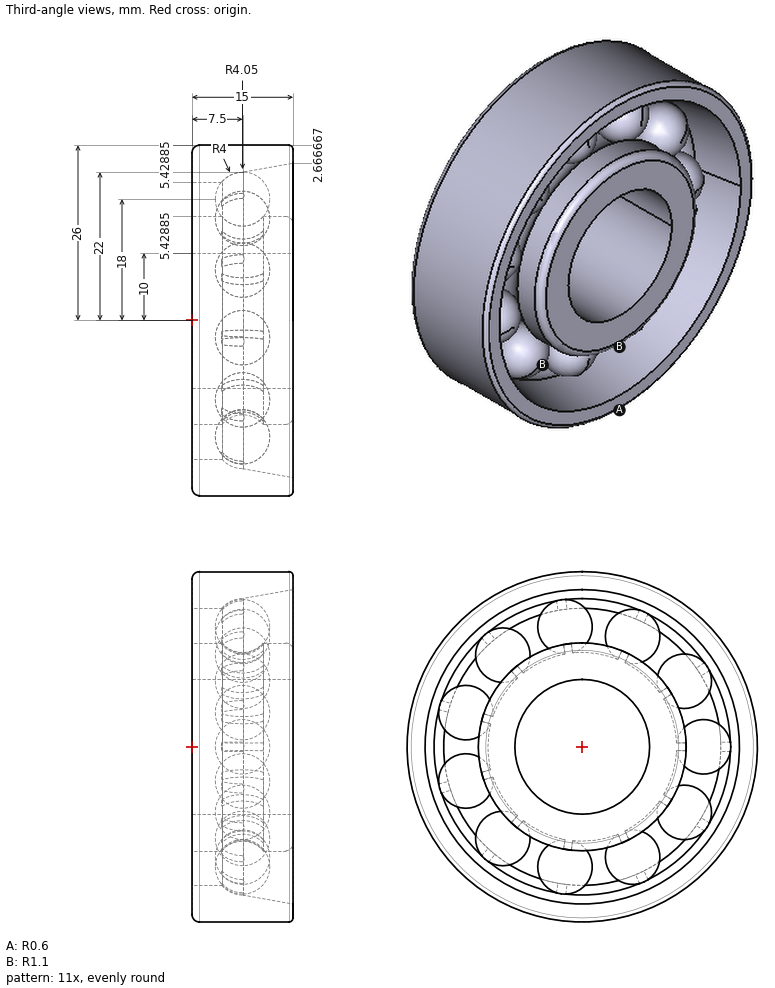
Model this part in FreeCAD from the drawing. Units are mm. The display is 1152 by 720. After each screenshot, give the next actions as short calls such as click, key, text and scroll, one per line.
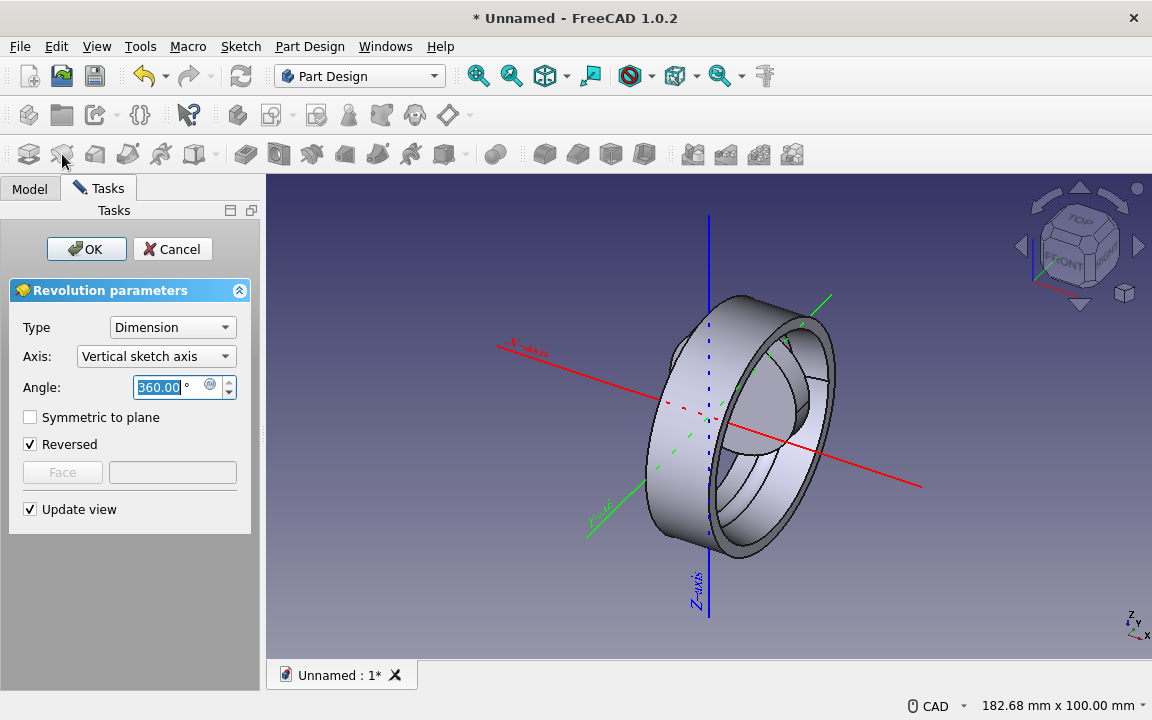
click(157, 356)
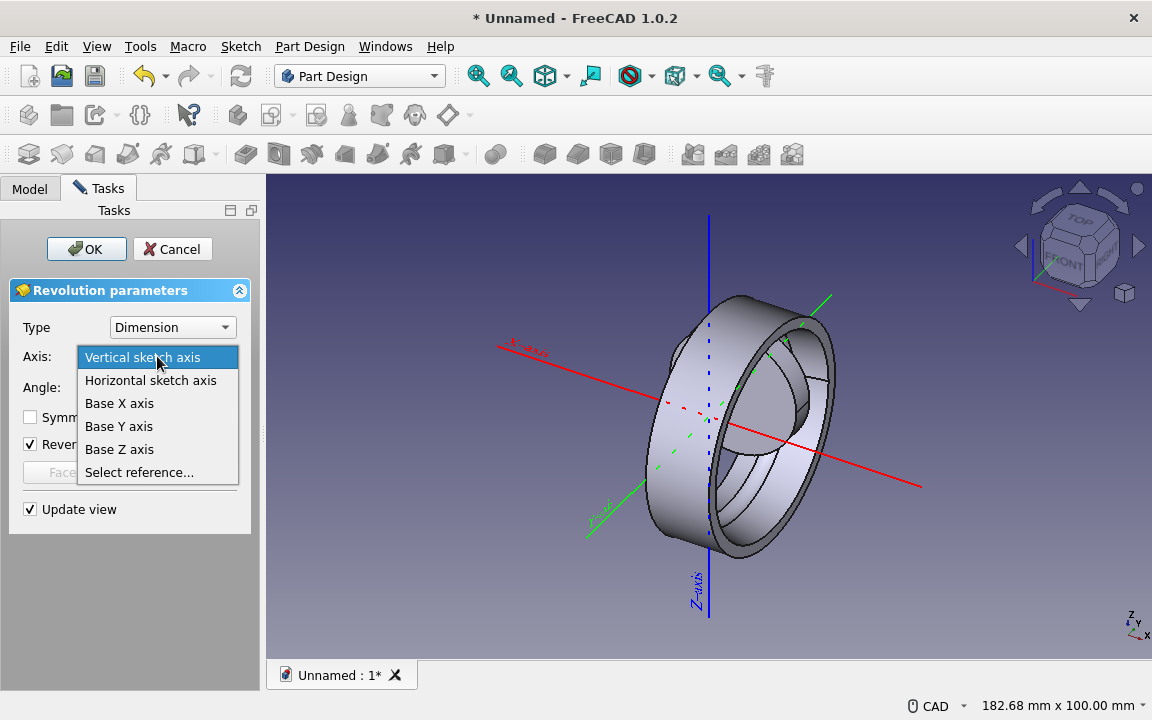
click(156, 380)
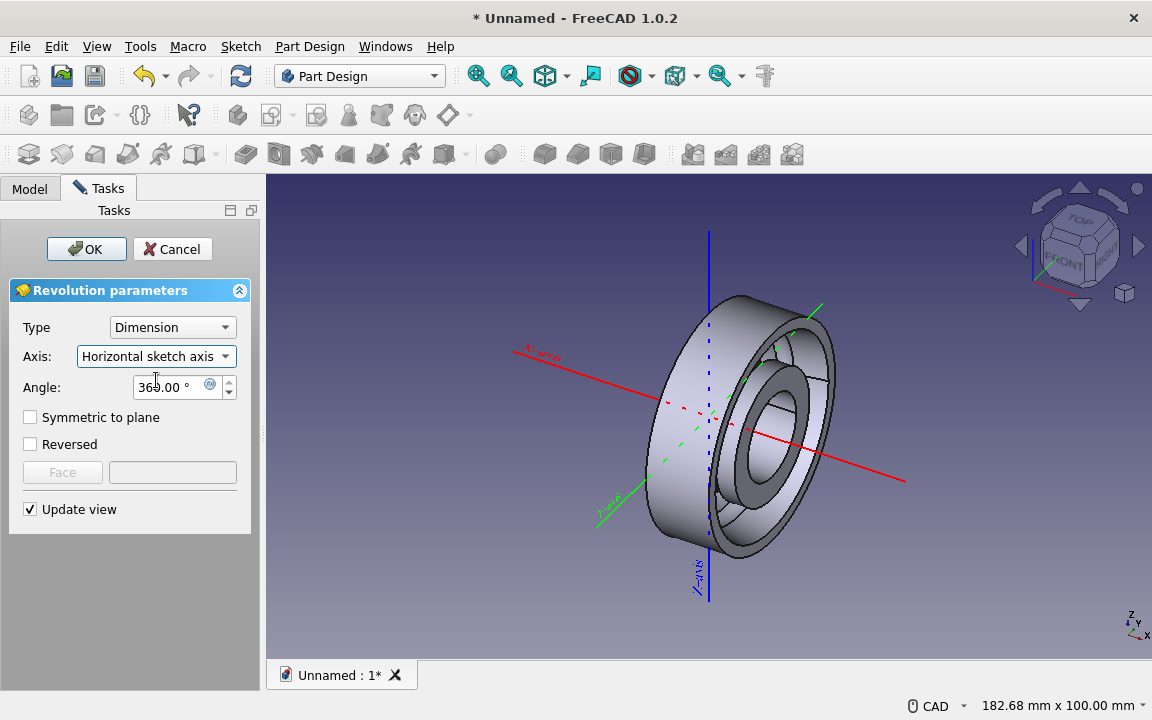
click(87, 249)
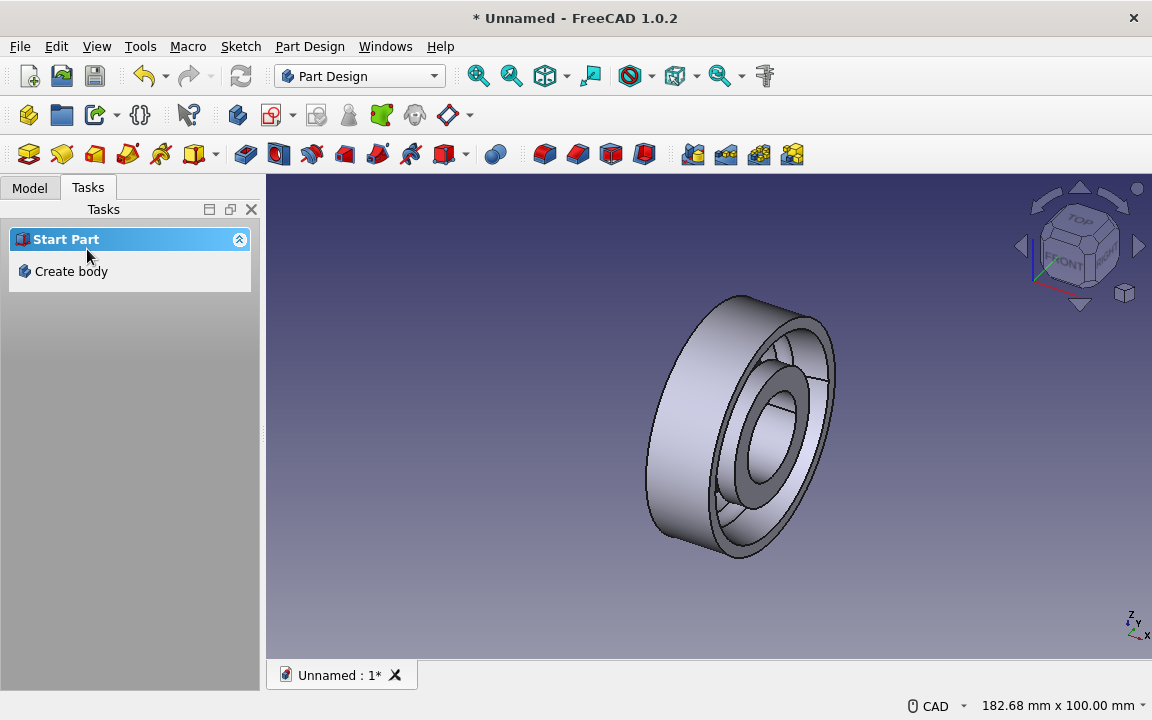
click(709, 499)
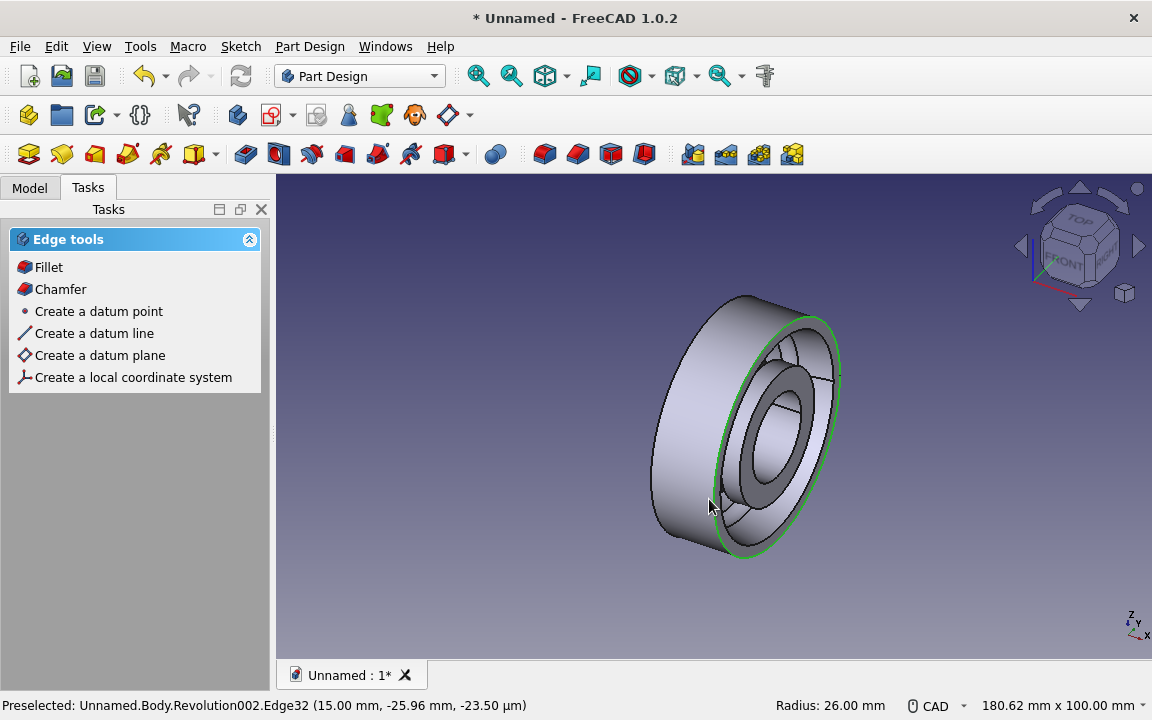
click(545, 154)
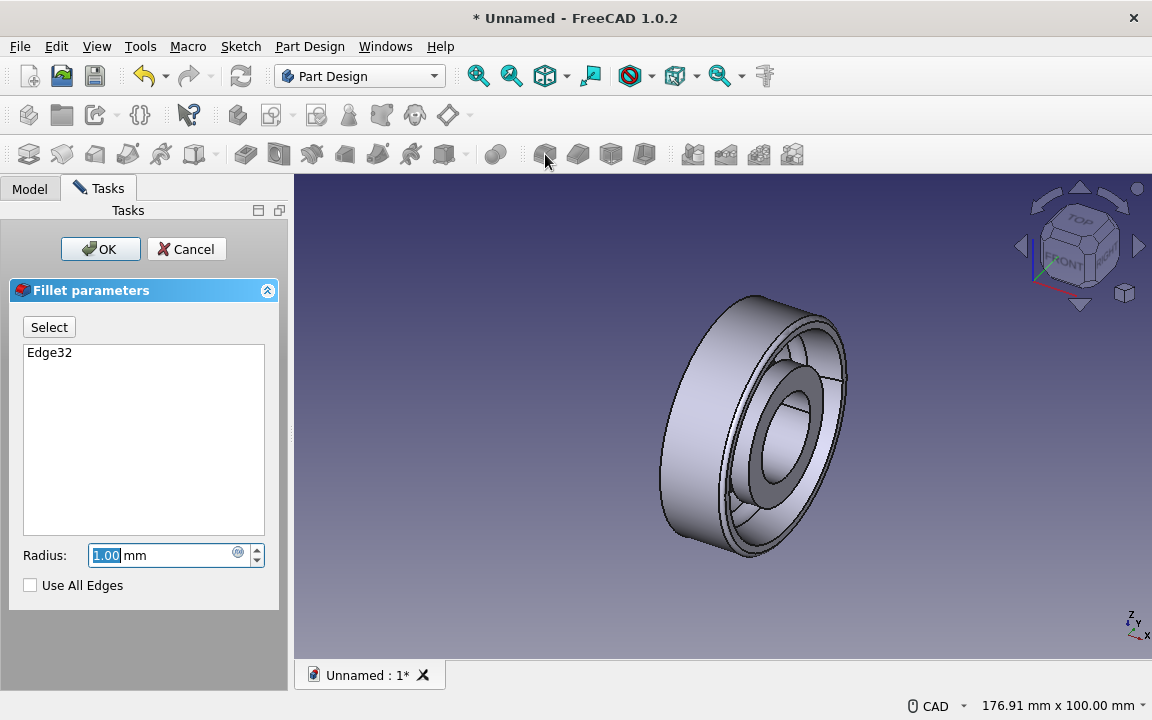
text(0.6)
key(Tab)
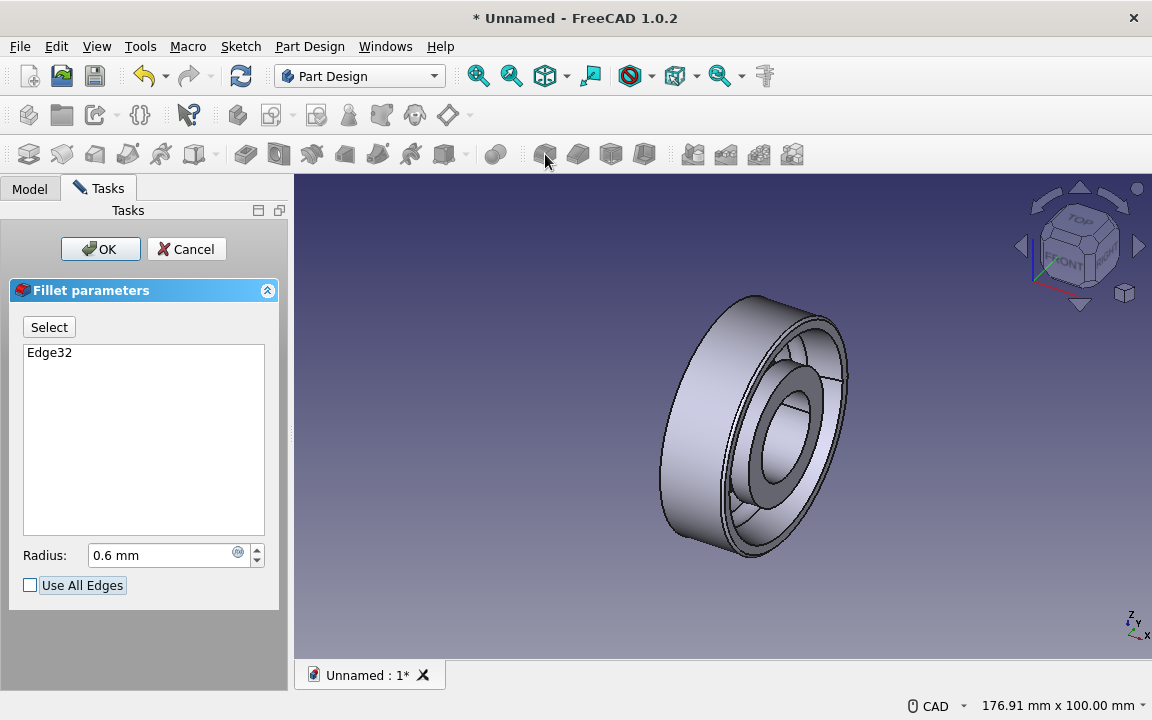
click(101, 249)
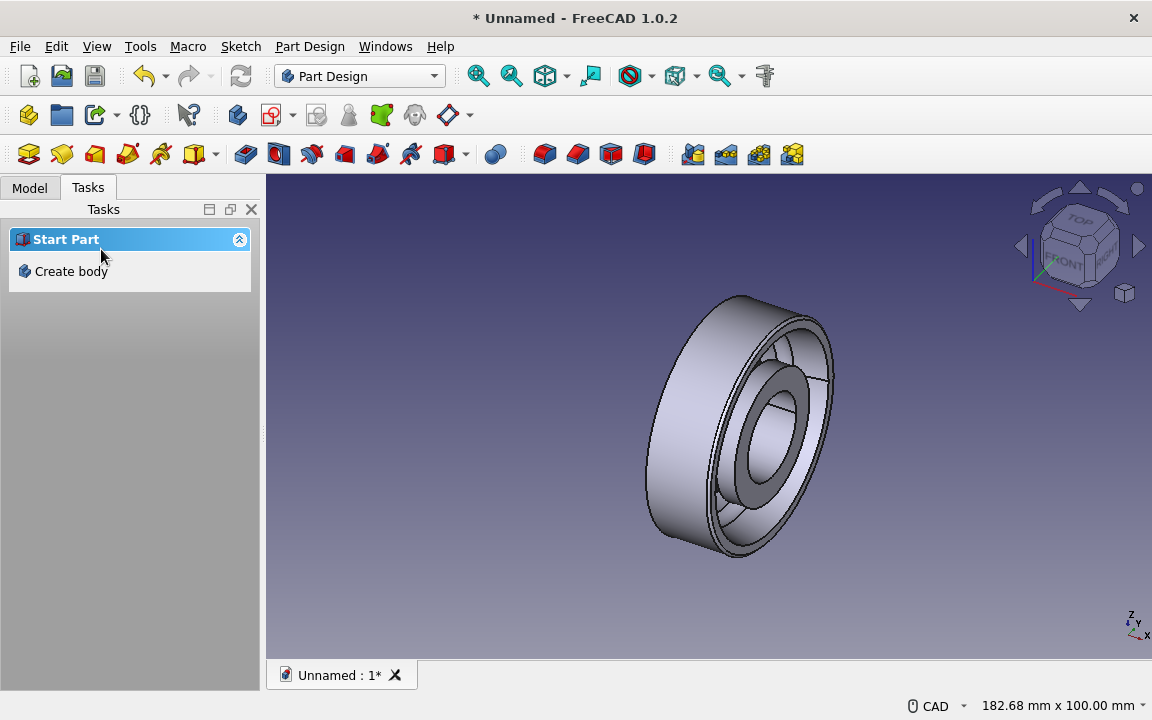
click(735, 474)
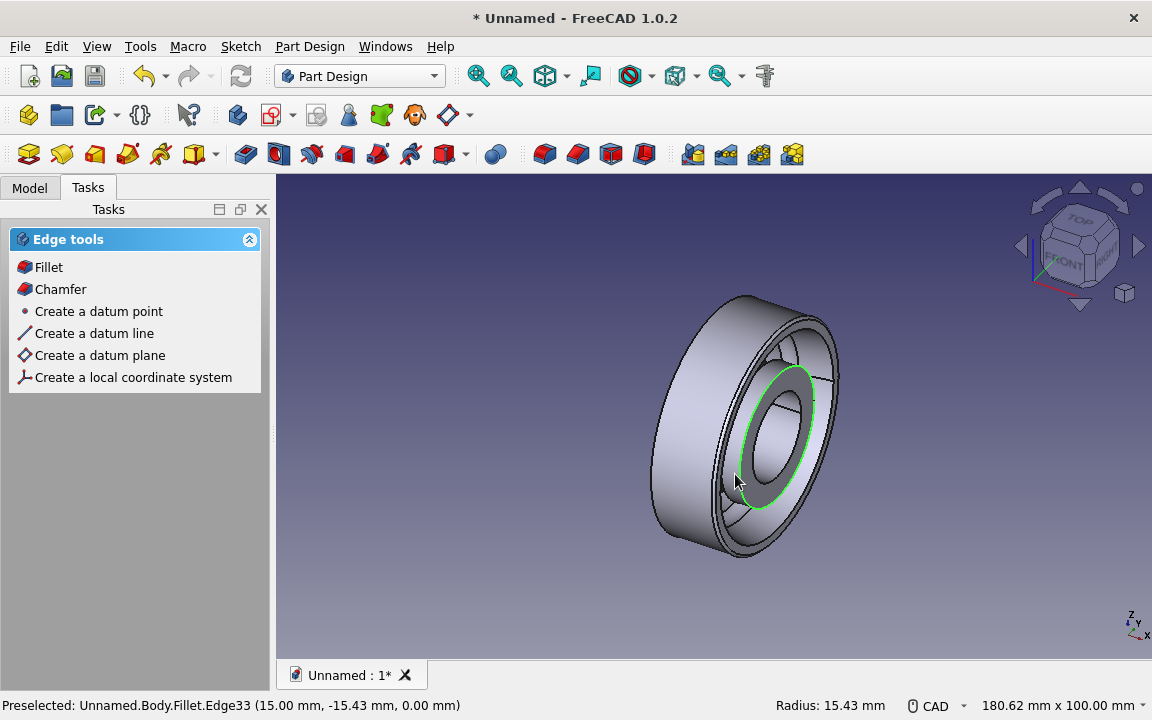
key(0)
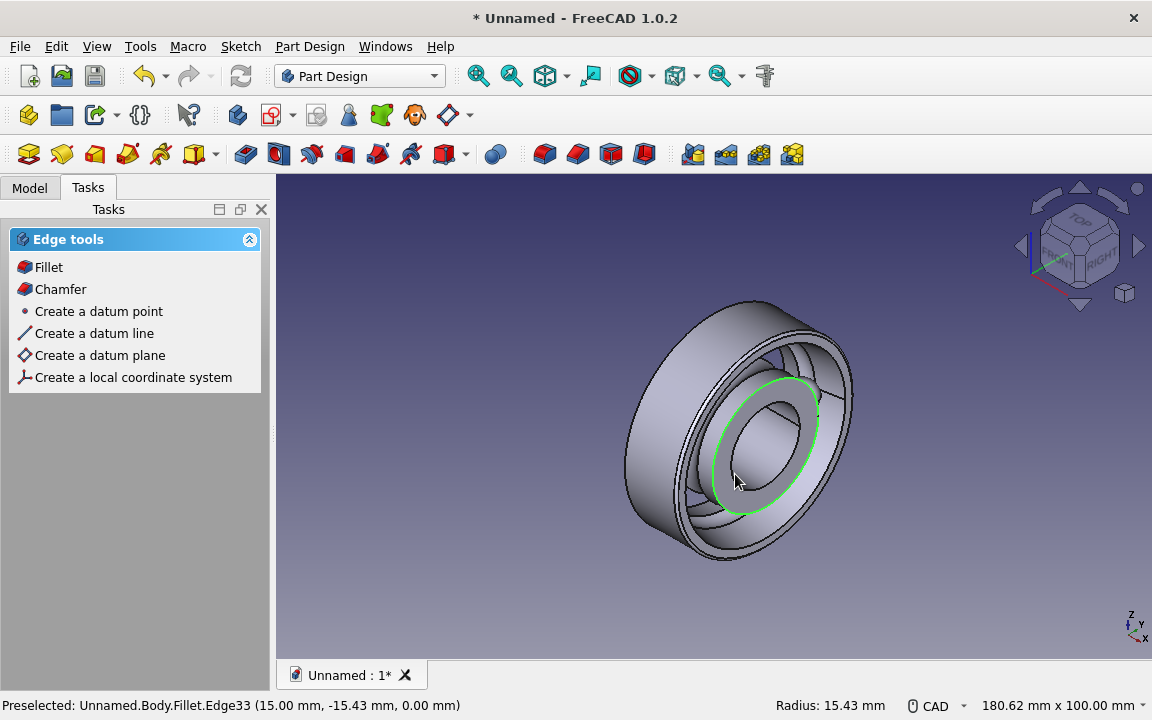
key(2)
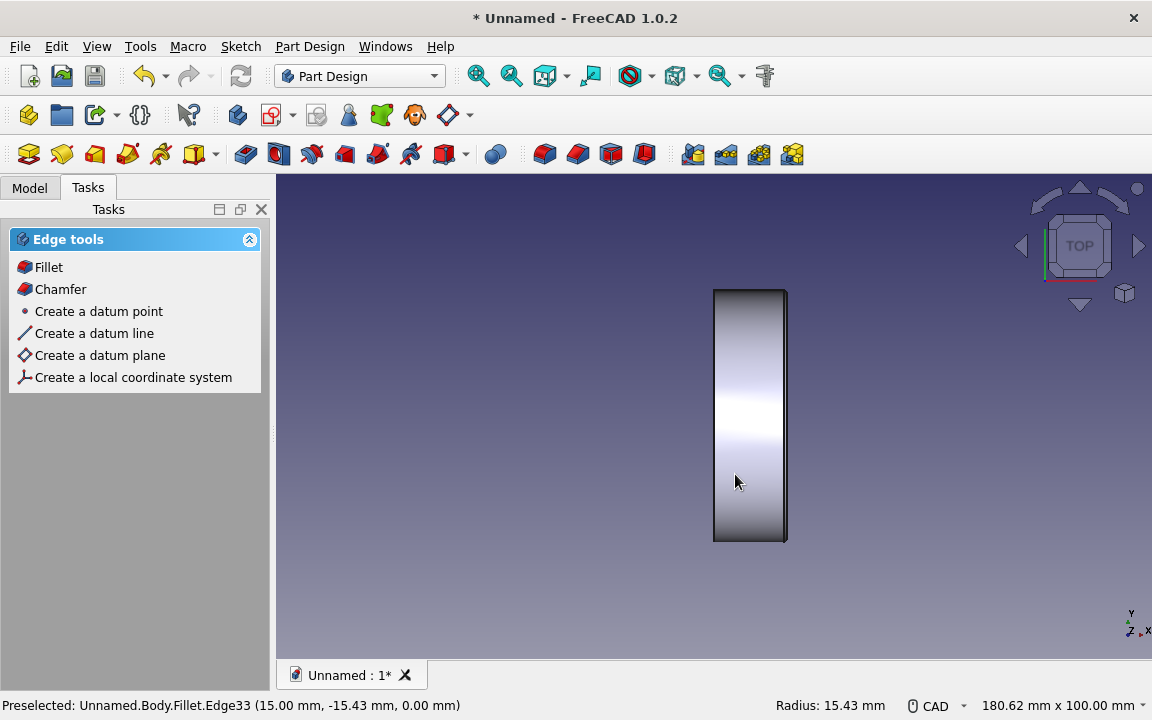
click(714, 324, ctrl)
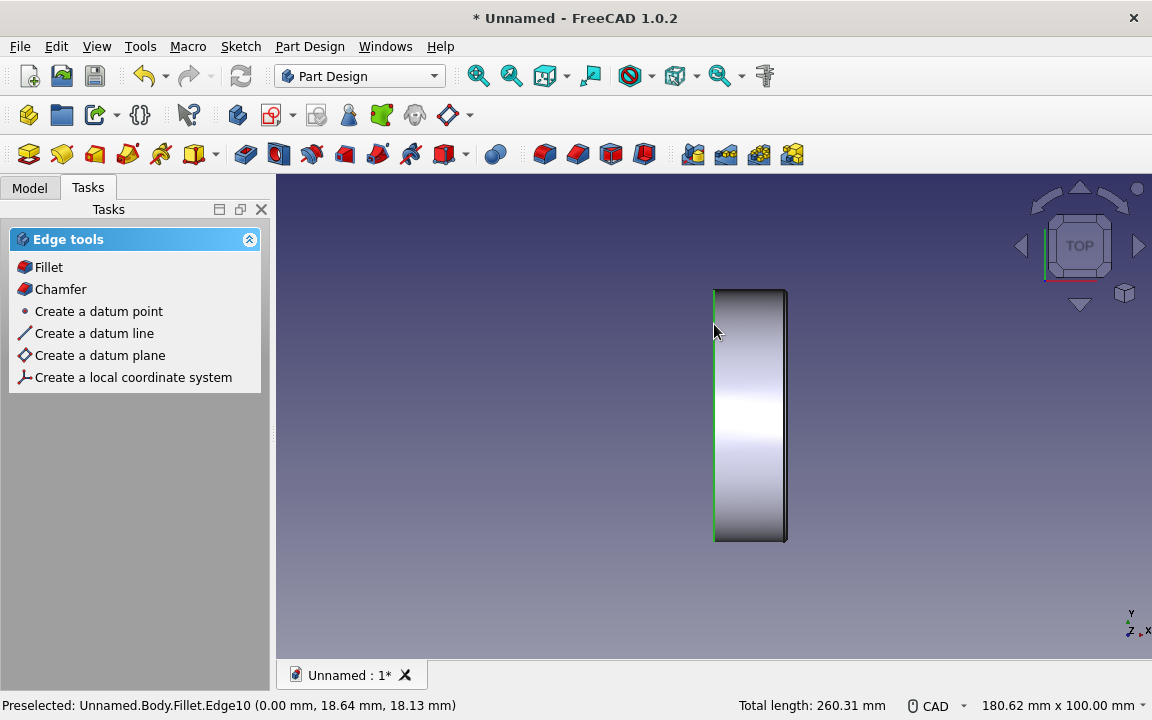
click(545, 154)